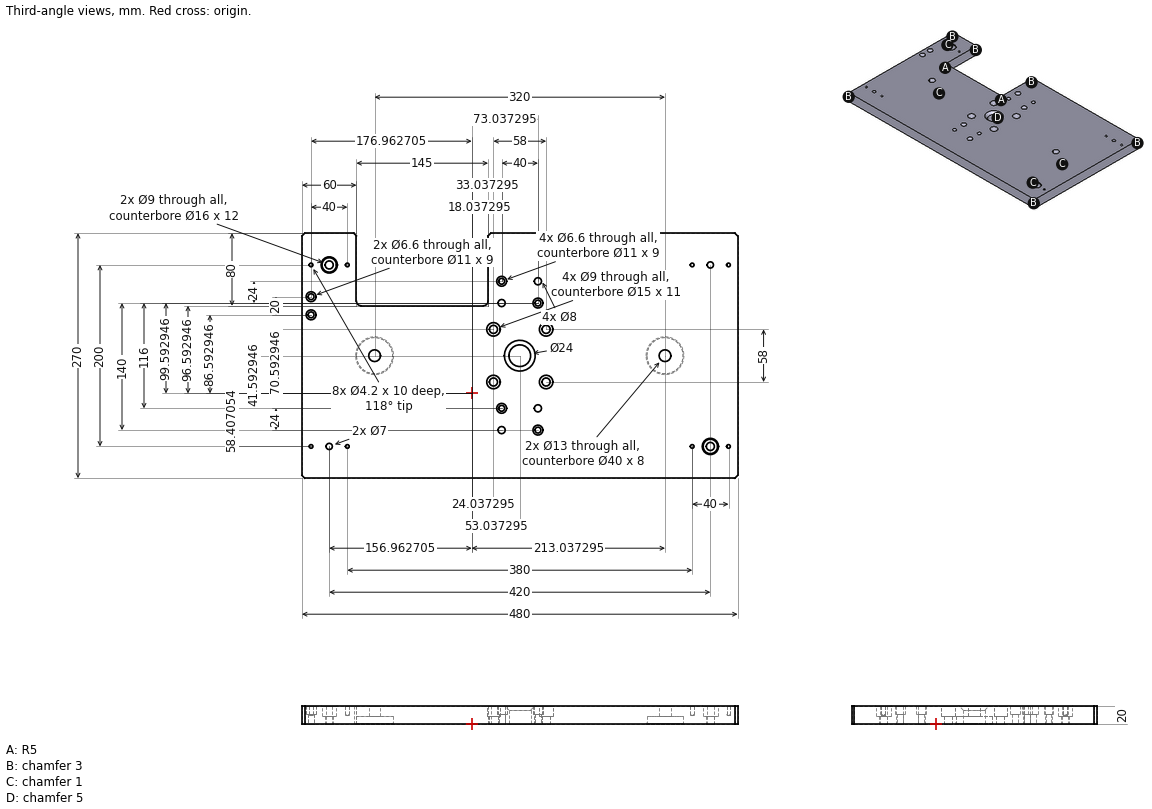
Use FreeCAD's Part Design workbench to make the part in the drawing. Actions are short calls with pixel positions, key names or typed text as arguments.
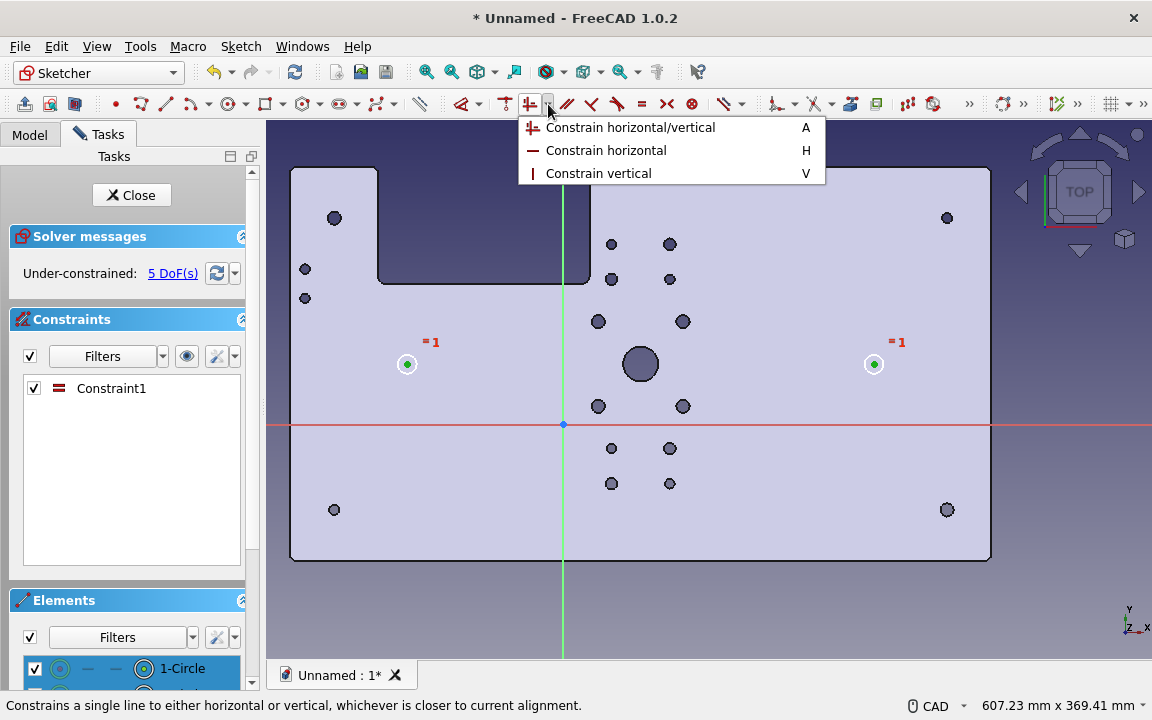
click(672, 150)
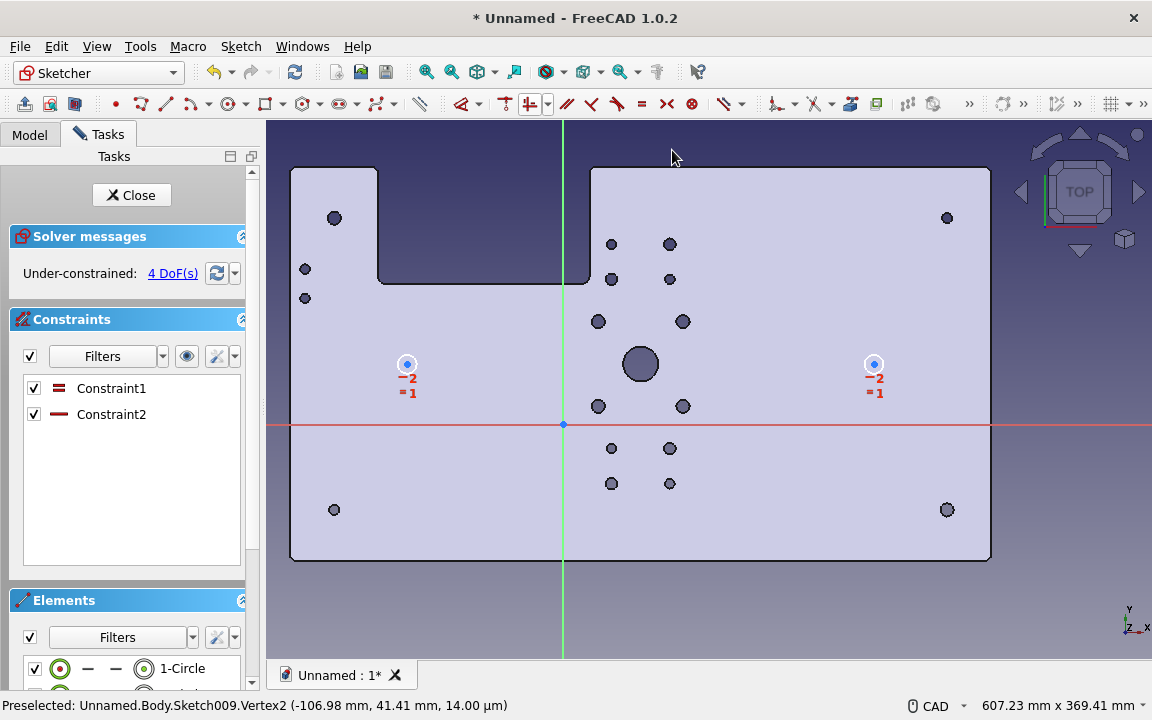
key(d)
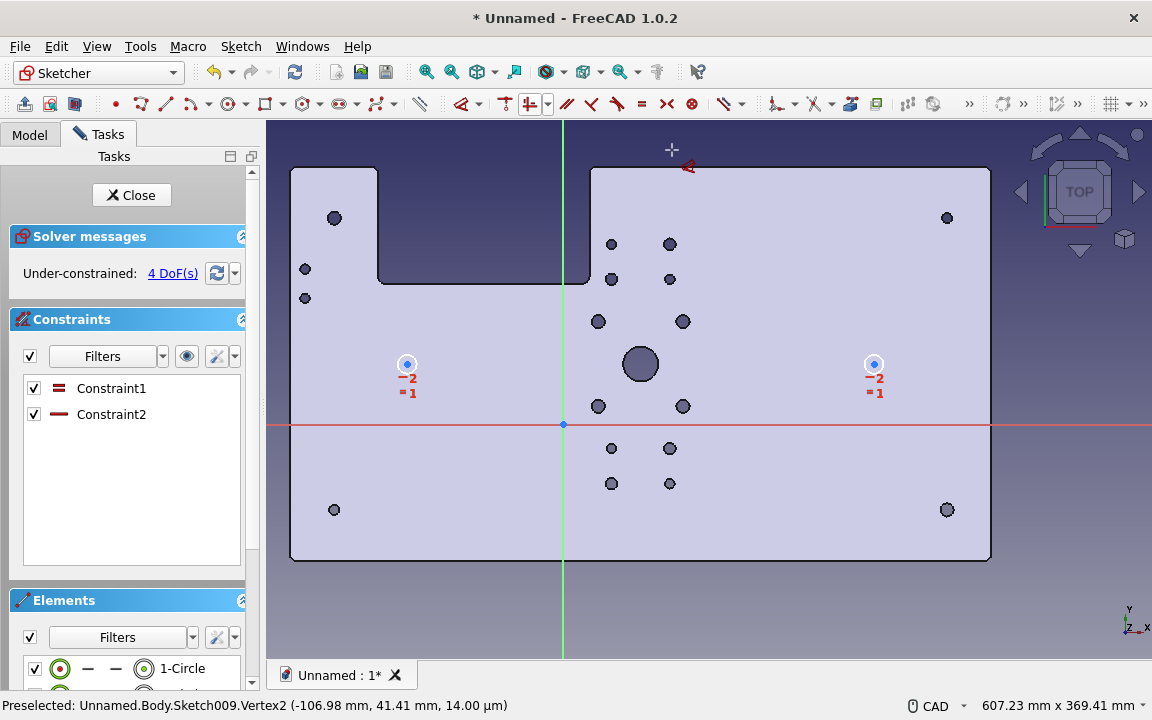
scroll(881, 358, up, 4)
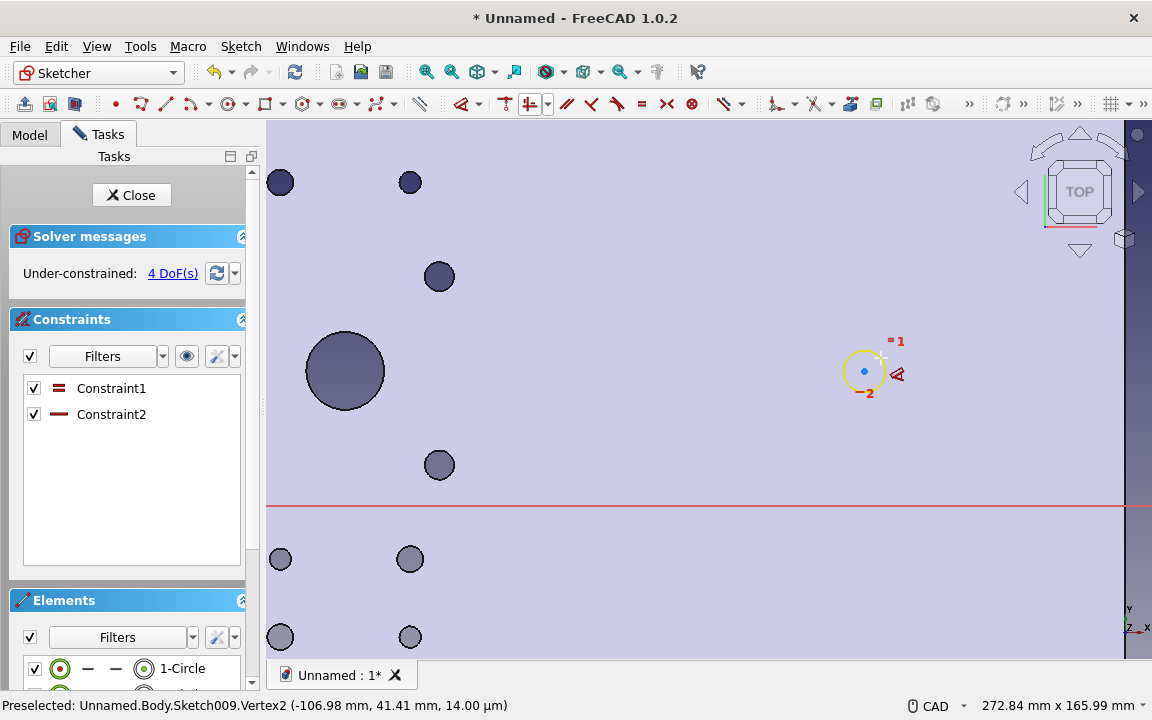
click(879, 357)
click(902, 334)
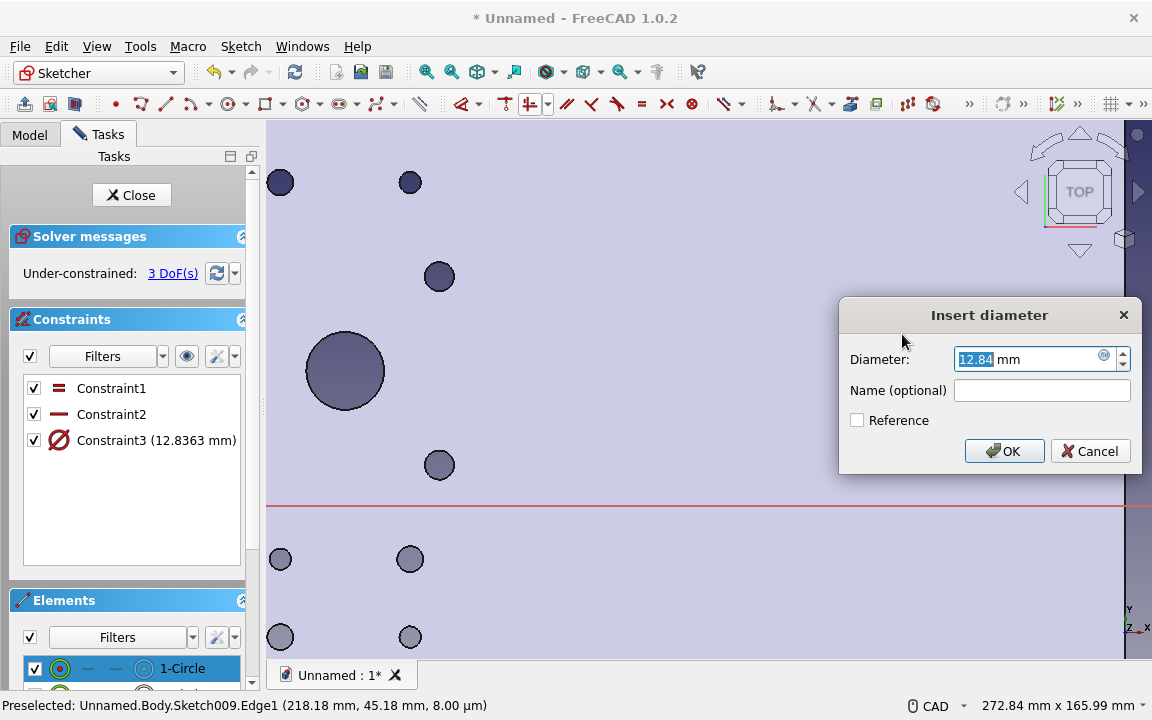
text(13)
key(Return)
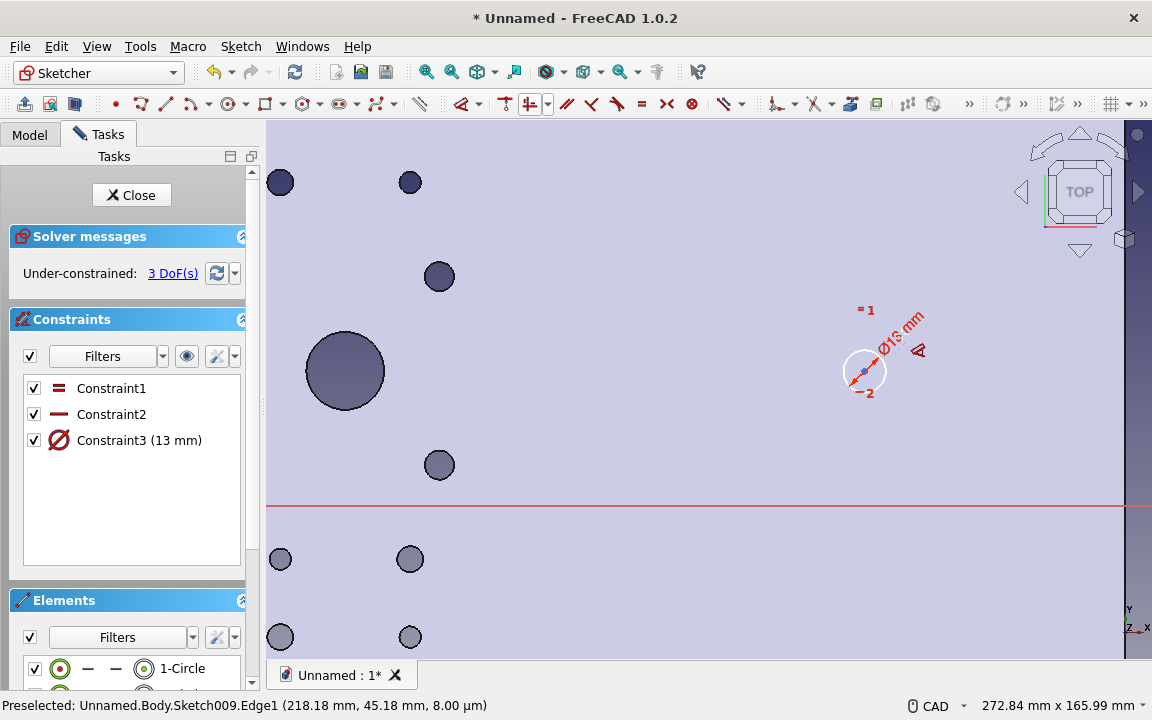
click(865, 371)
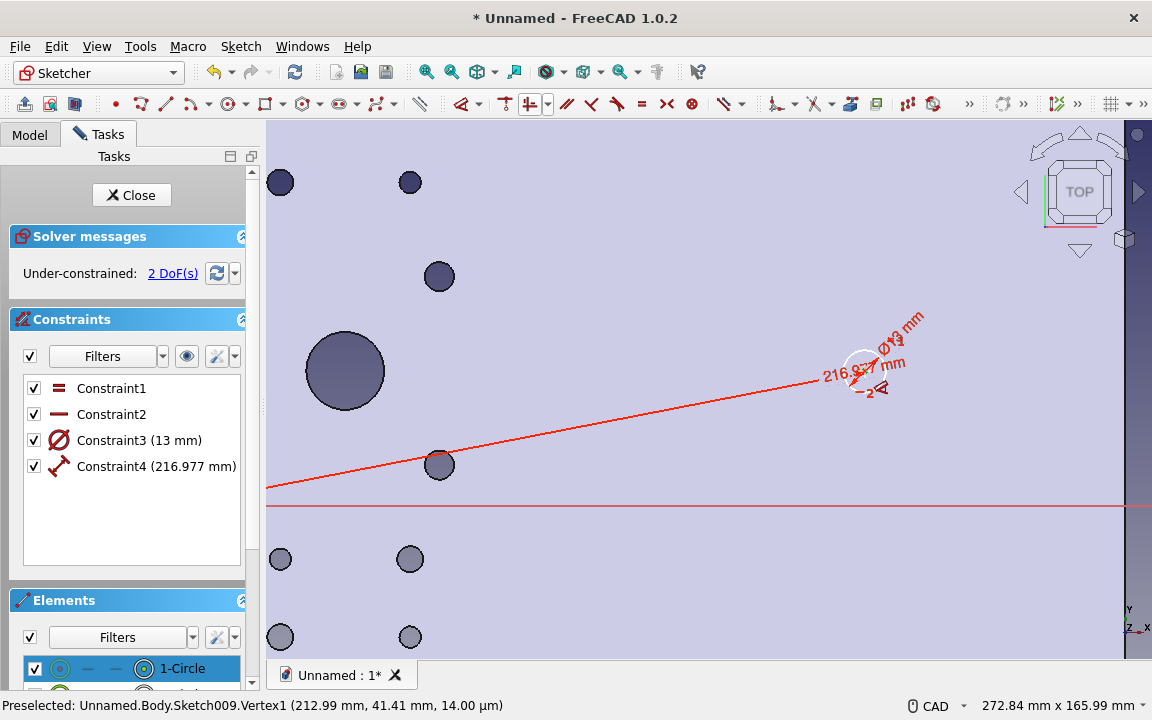
scroll(881, 358, down, 4)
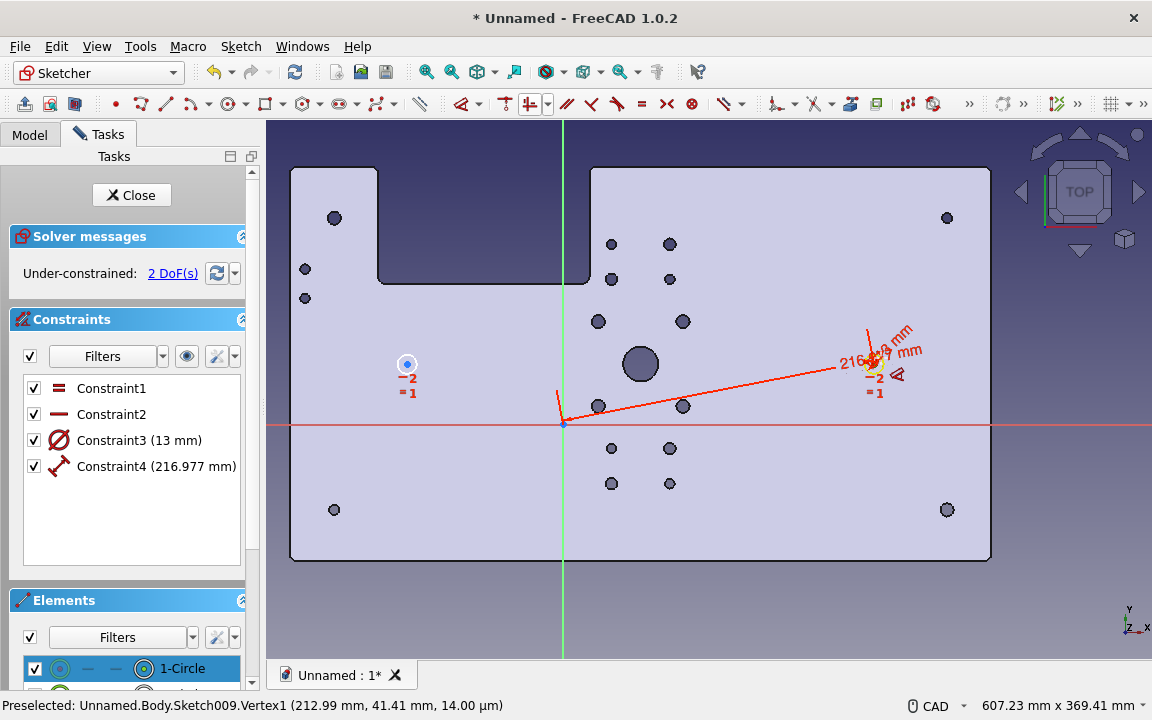
click(407, 364)
click(641, 330)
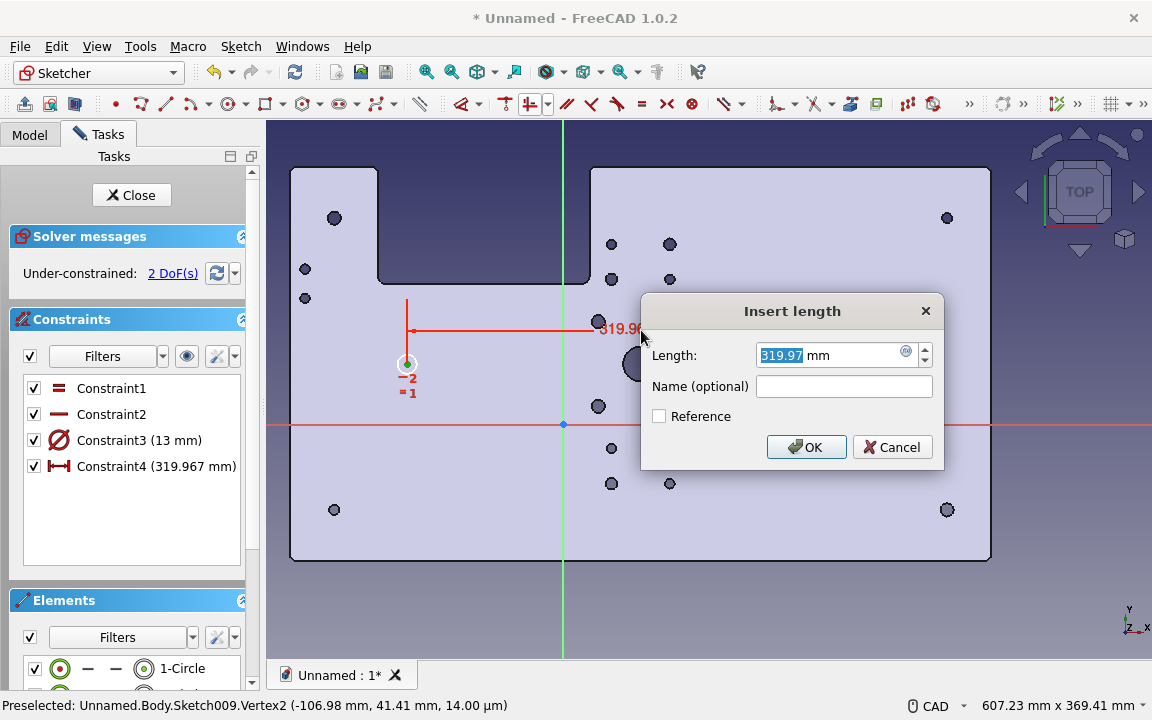
text(320)
key(Return)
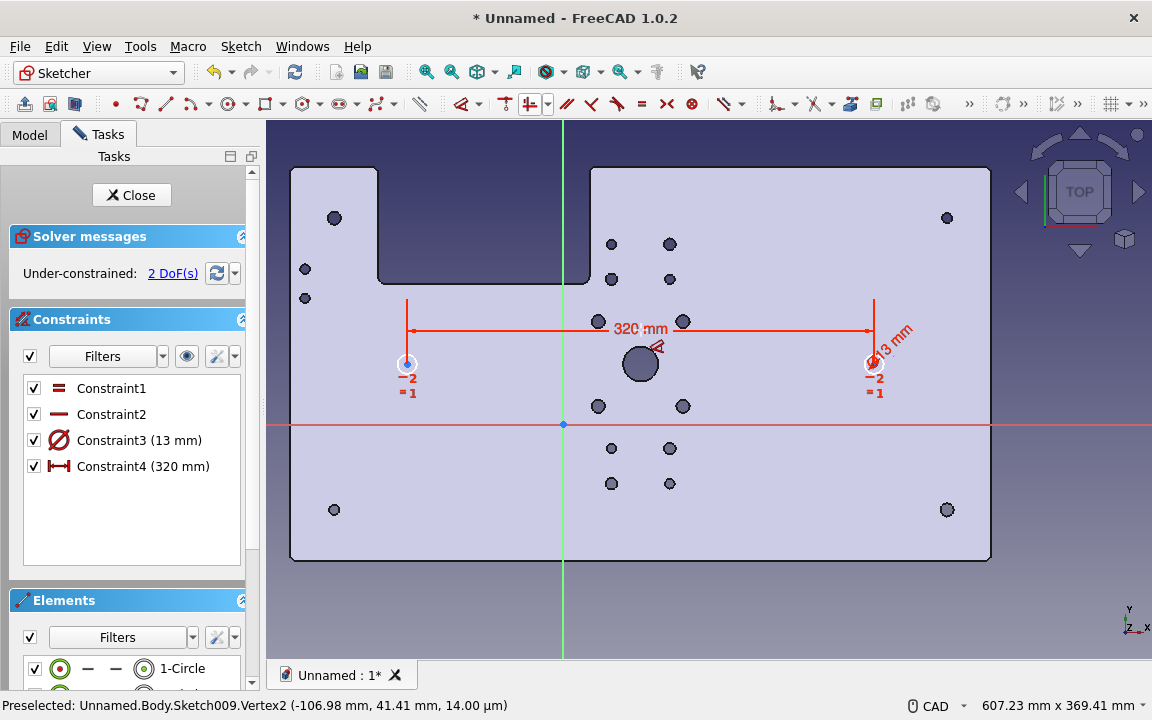
click(874, 364)
click(908, 394)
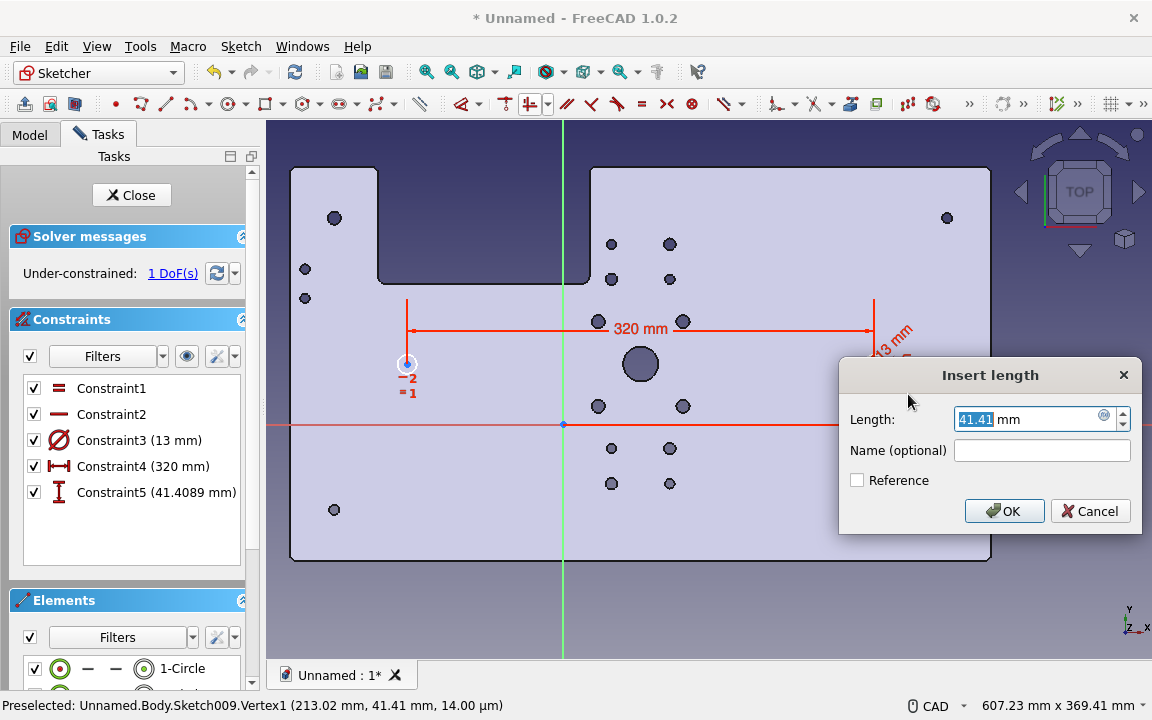
text(41.592946)
key(Return)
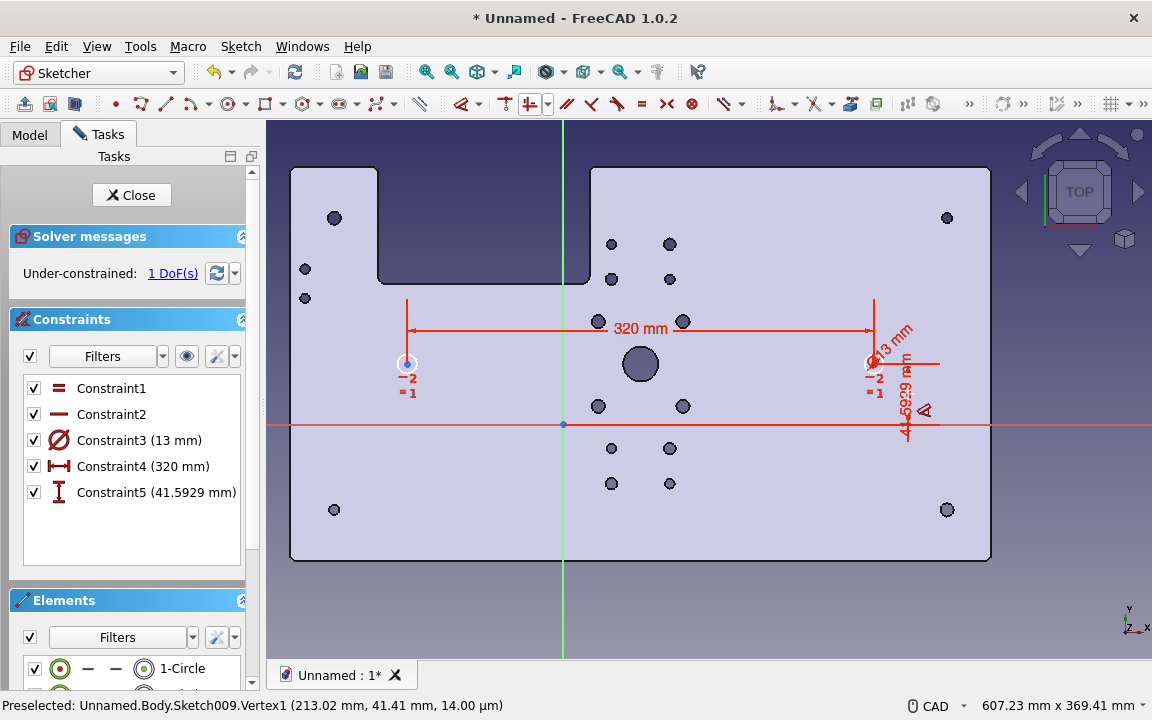
click(874, 364)
click(719, 459)